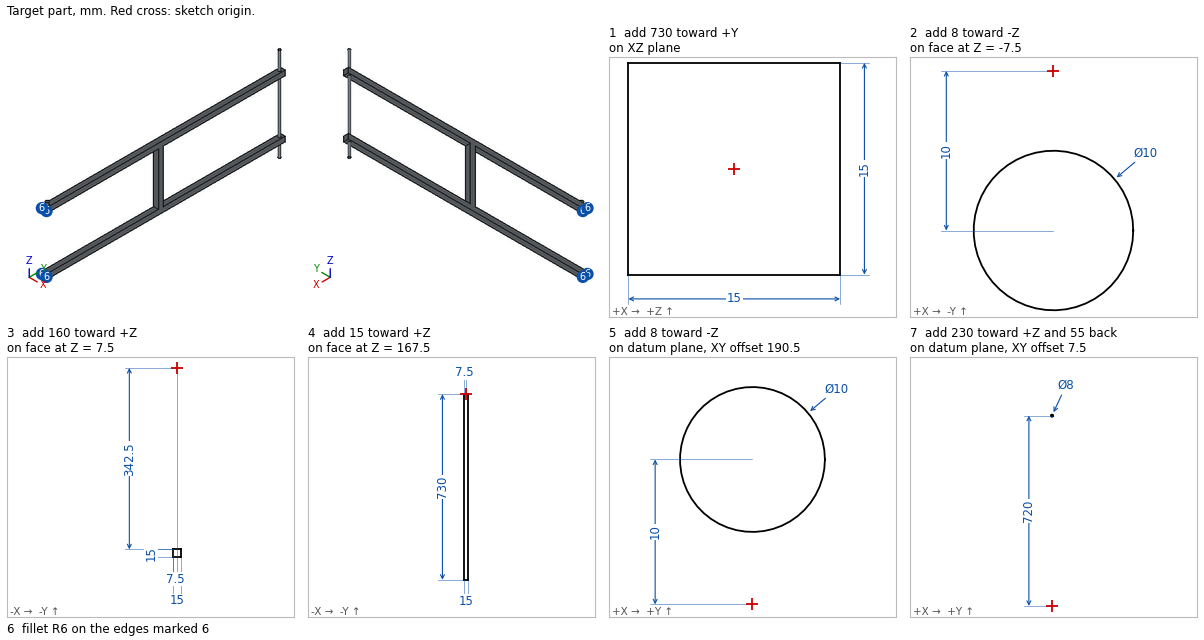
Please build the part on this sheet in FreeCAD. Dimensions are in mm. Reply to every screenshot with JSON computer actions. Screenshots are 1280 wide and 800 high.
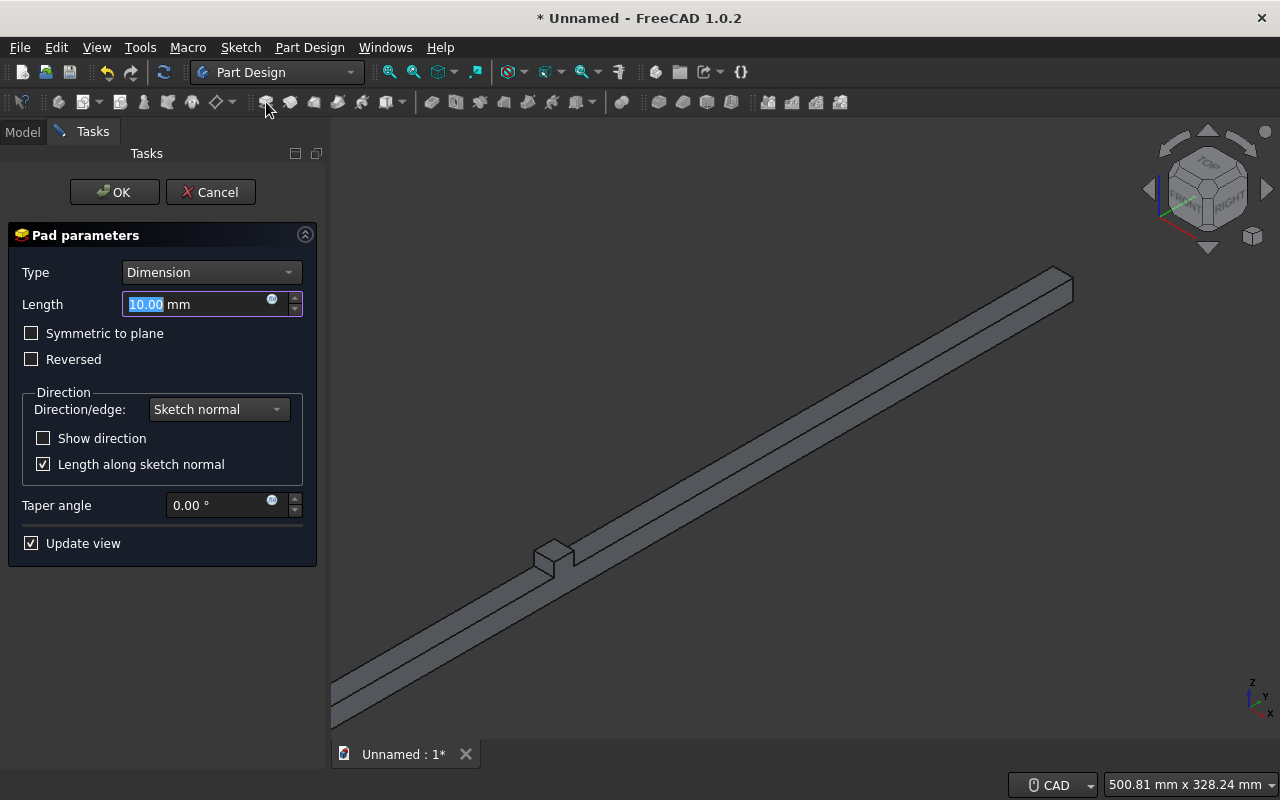
{"action": "type", "text": "160"}
{"action": "key", "text": "Tab"}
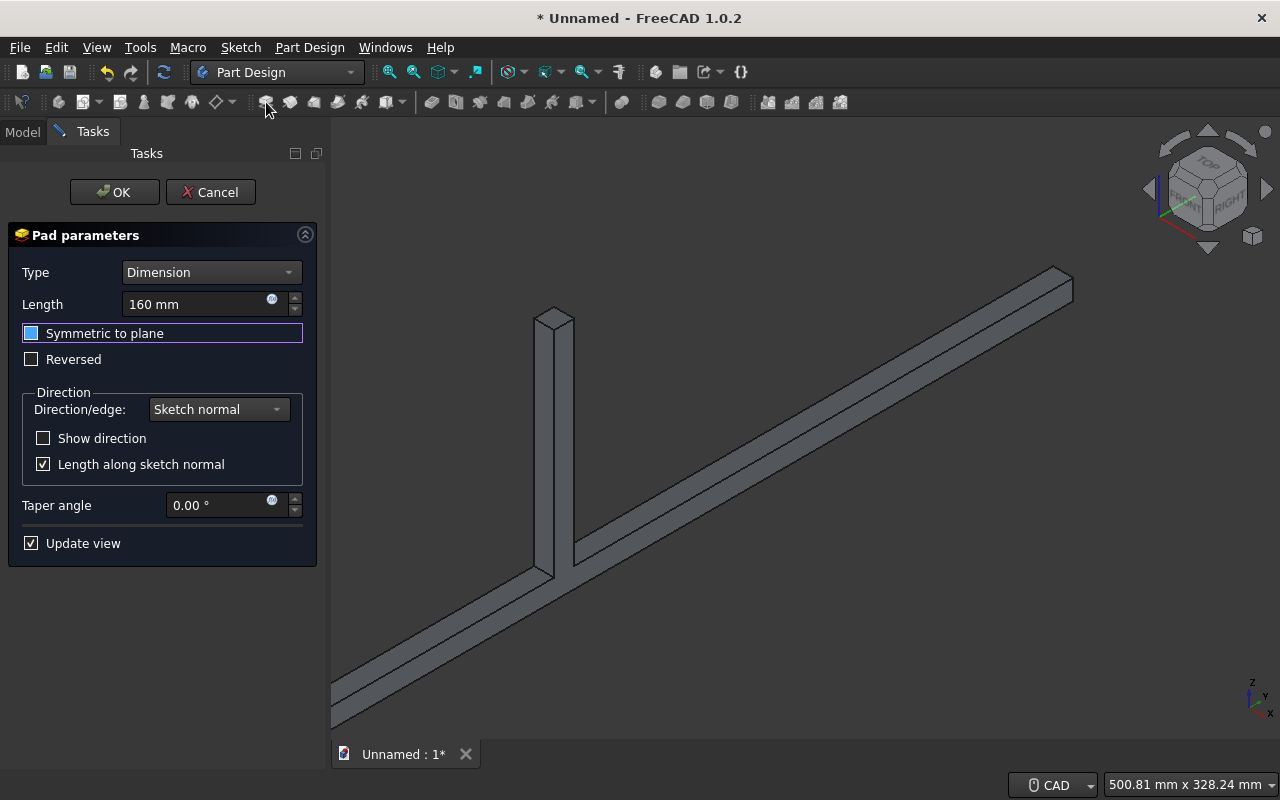
{"action": "left_click", "coordinate": [115, 192]}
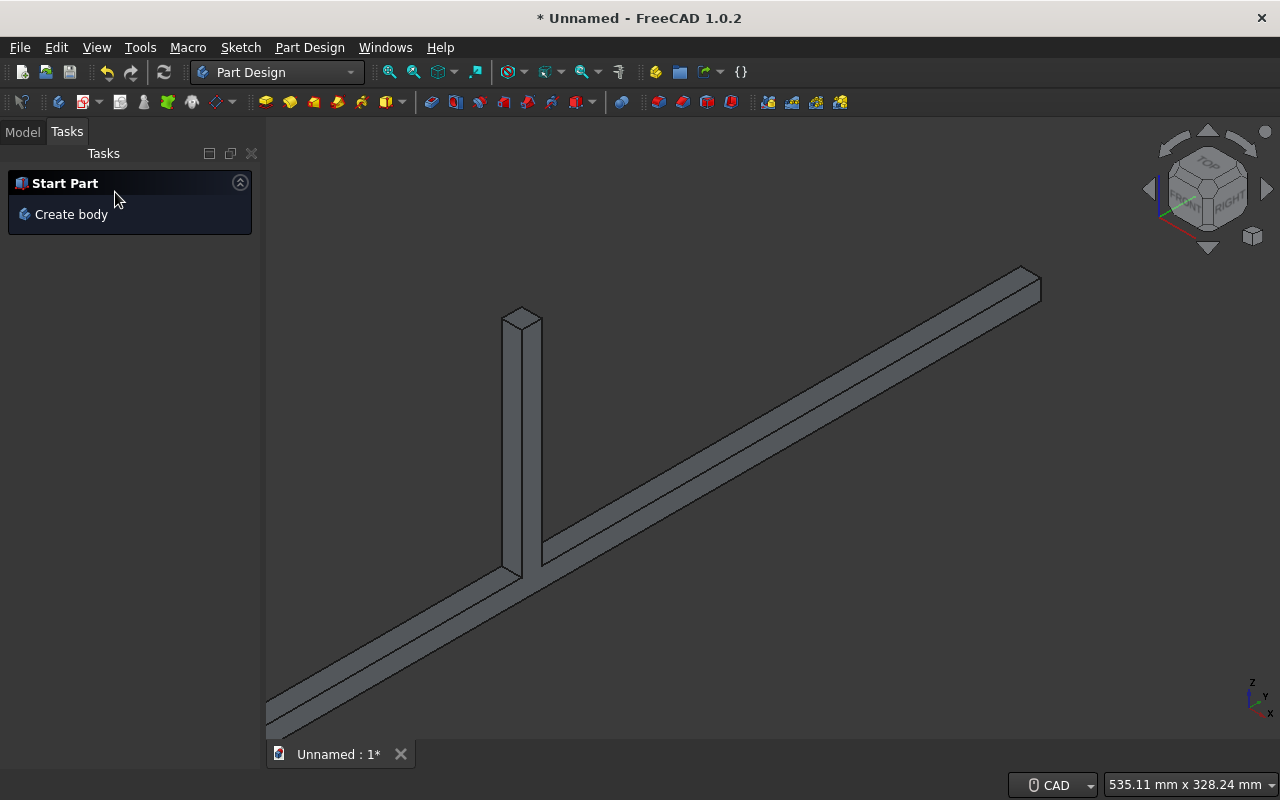
{"action": "left_click", "coordinate": [390, 72]}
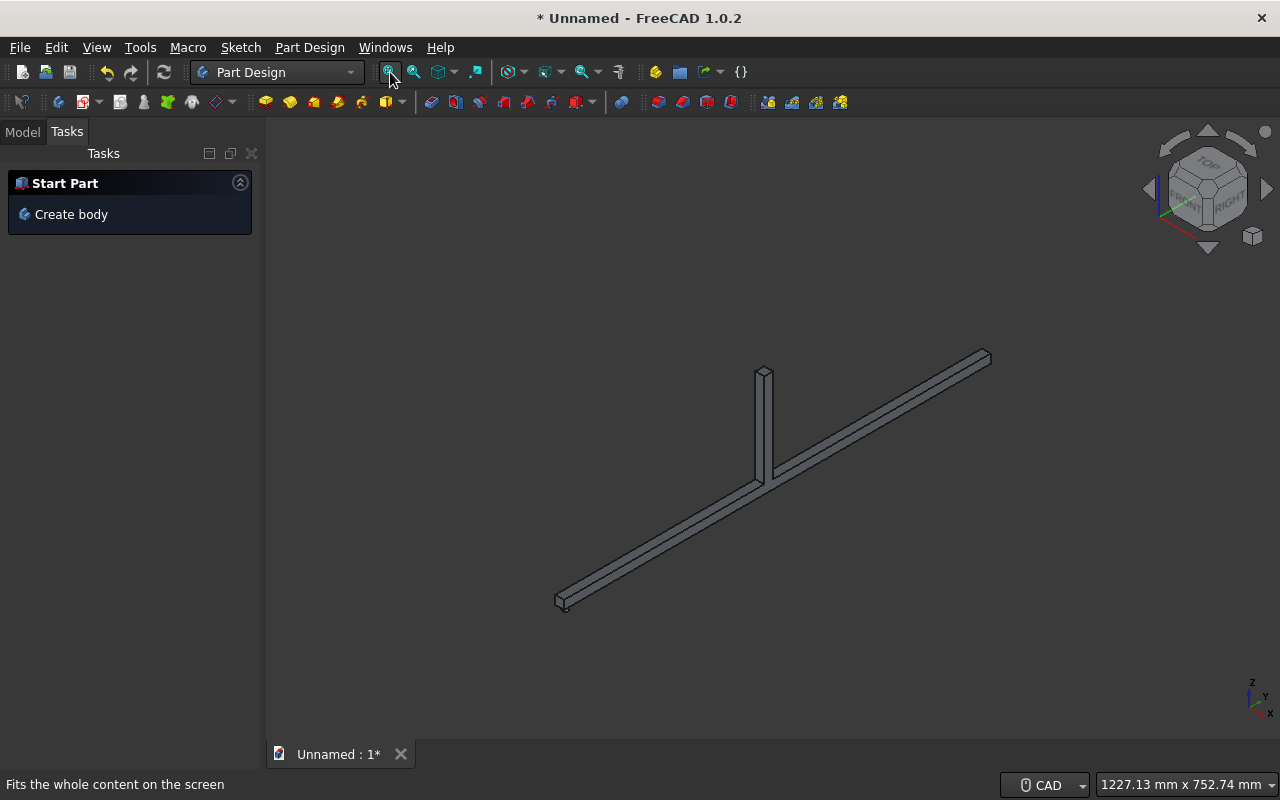
{"action": "scroll", "coordinate": [764, 370], "scroll_direction": "up", "scroll_amount": 4}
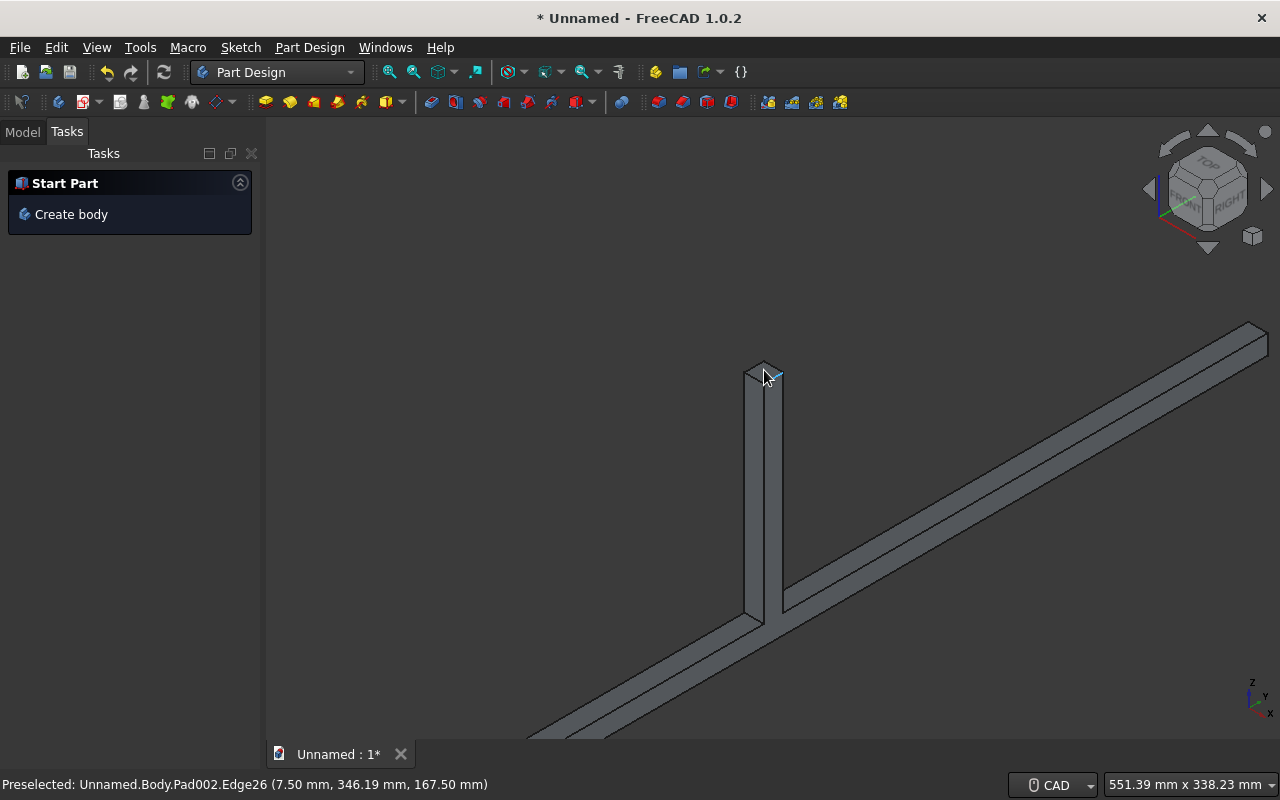
{"action": "left_click", "coordinate": [764, 371]}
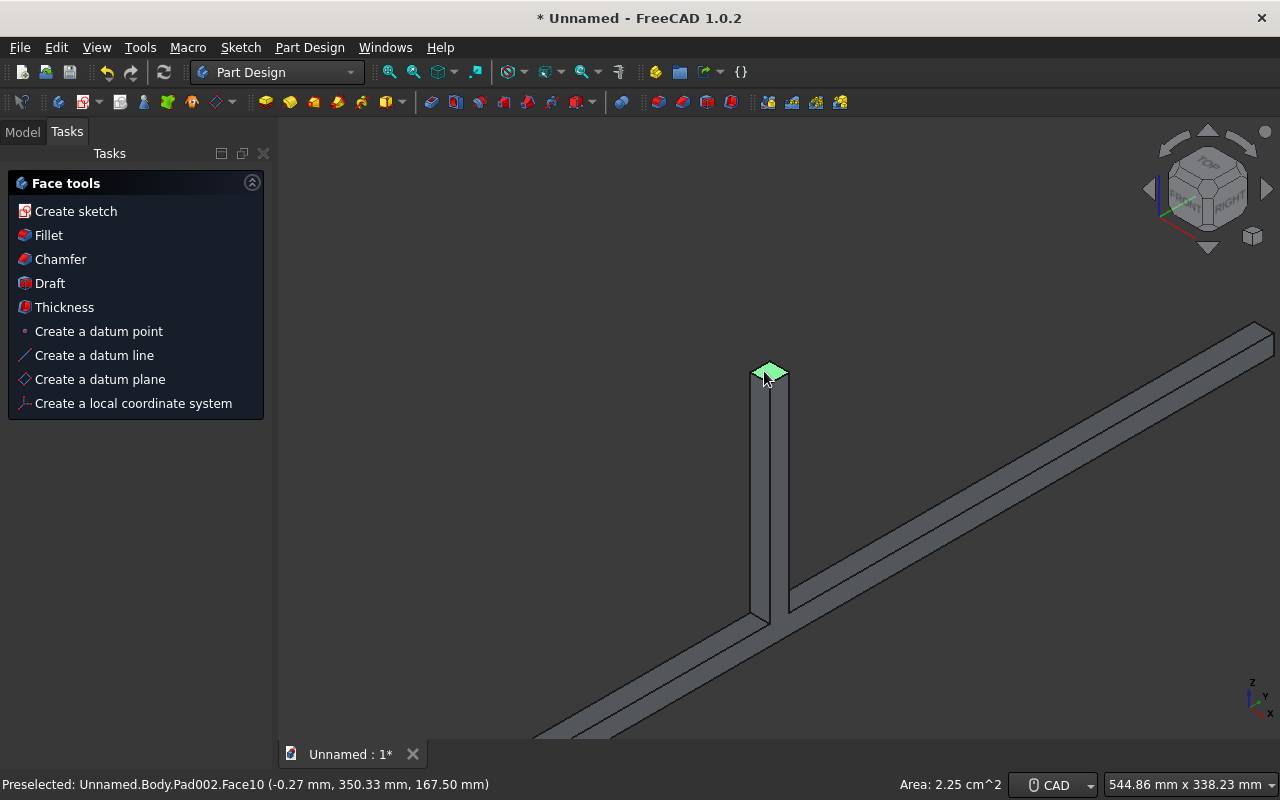
{"action": "left_click", "coordinate": [84, 102]}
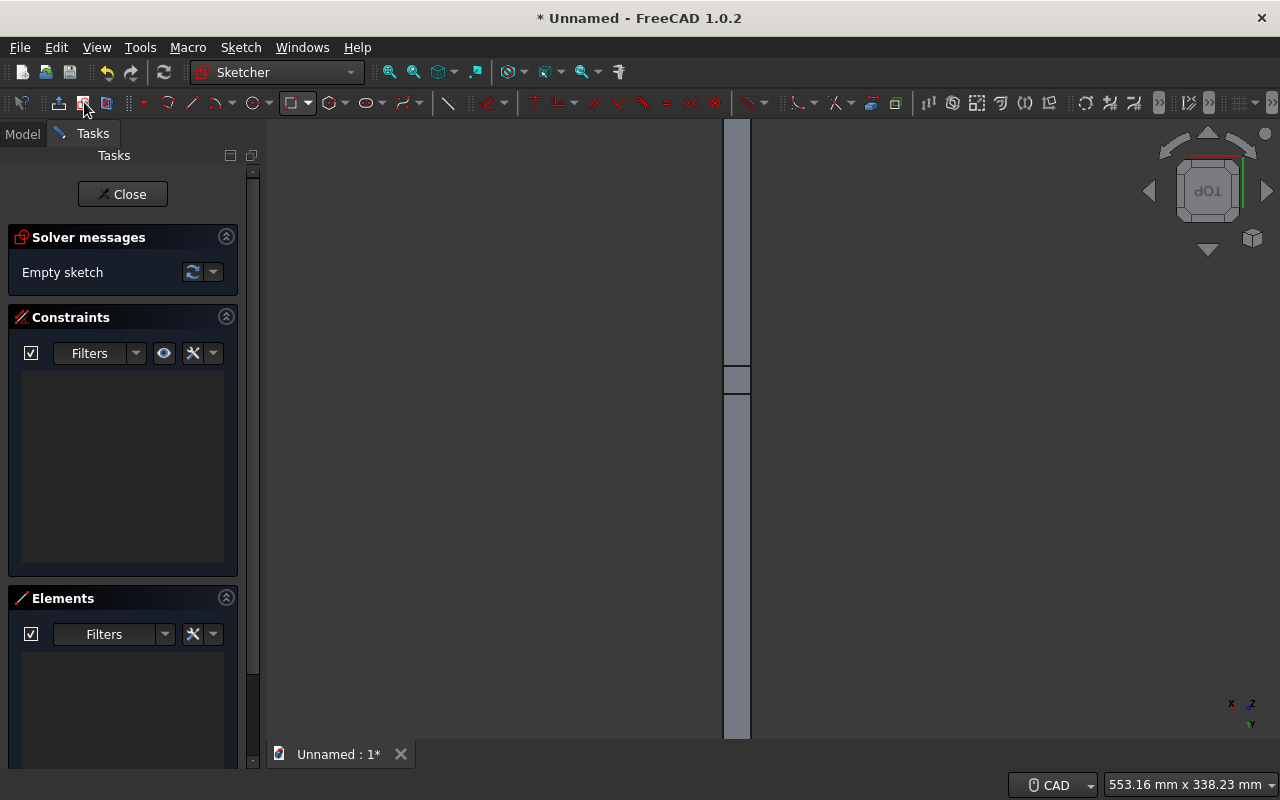
{"action": "scroll", "coordinate": [691, 438], "scroll_direction": "down", "scroll_amount": 6}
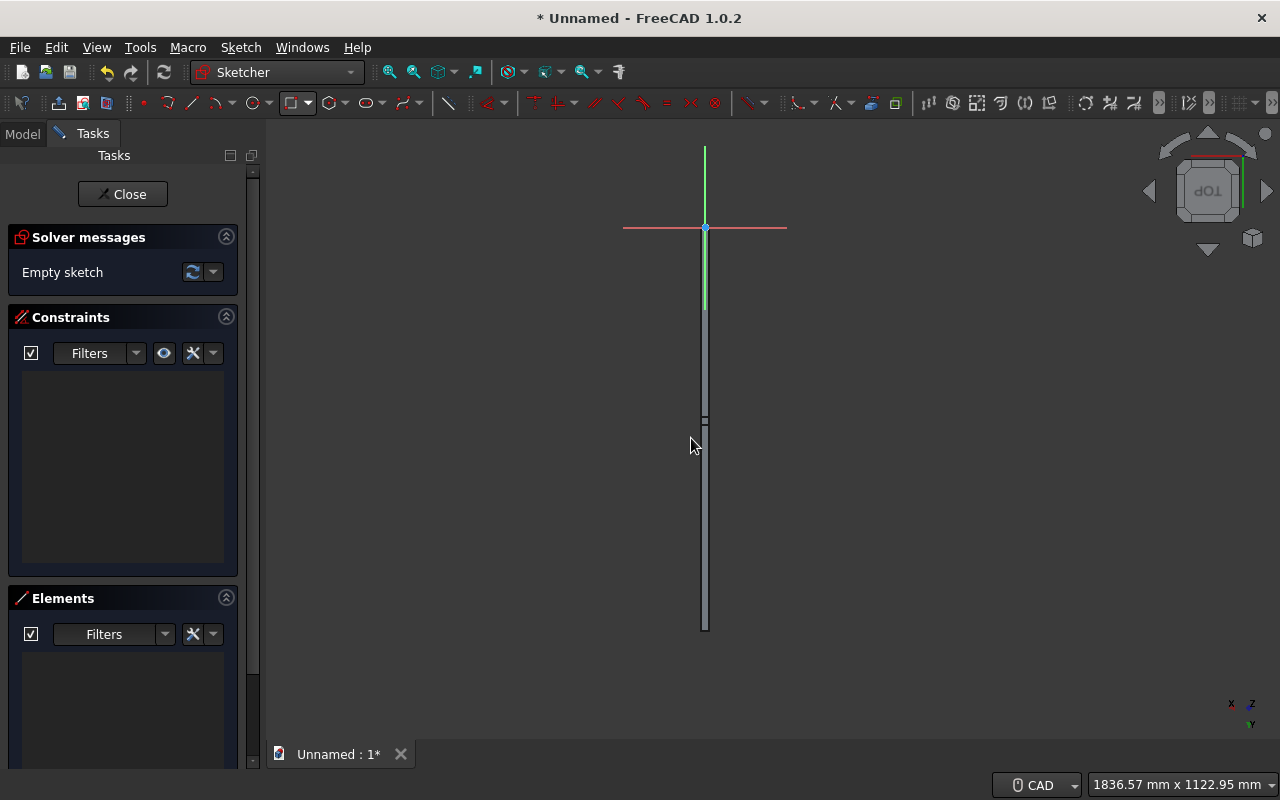
{"action": "left_click", "coordinate": [292, 104]}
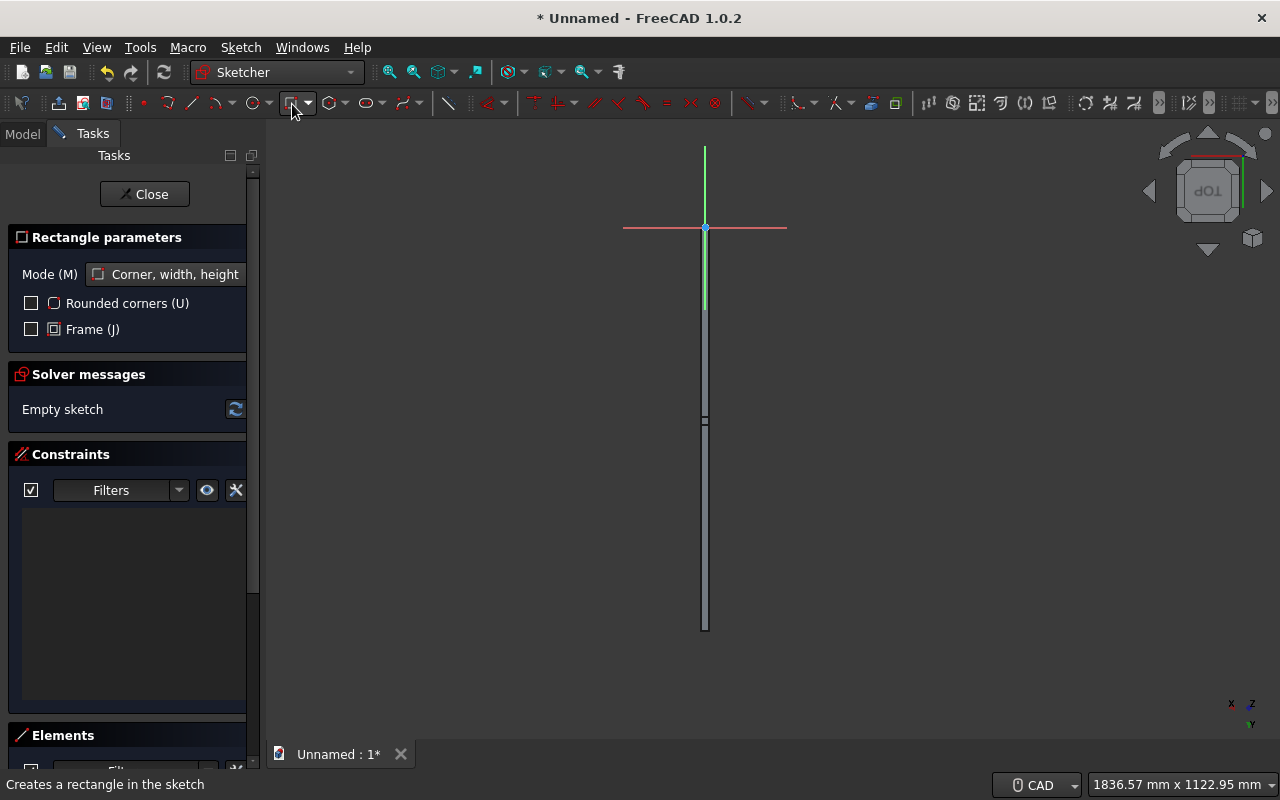
{"action": "scroll", "coordinate": [701, 228], "scroll_direction": "up", "scroll_amount": 7}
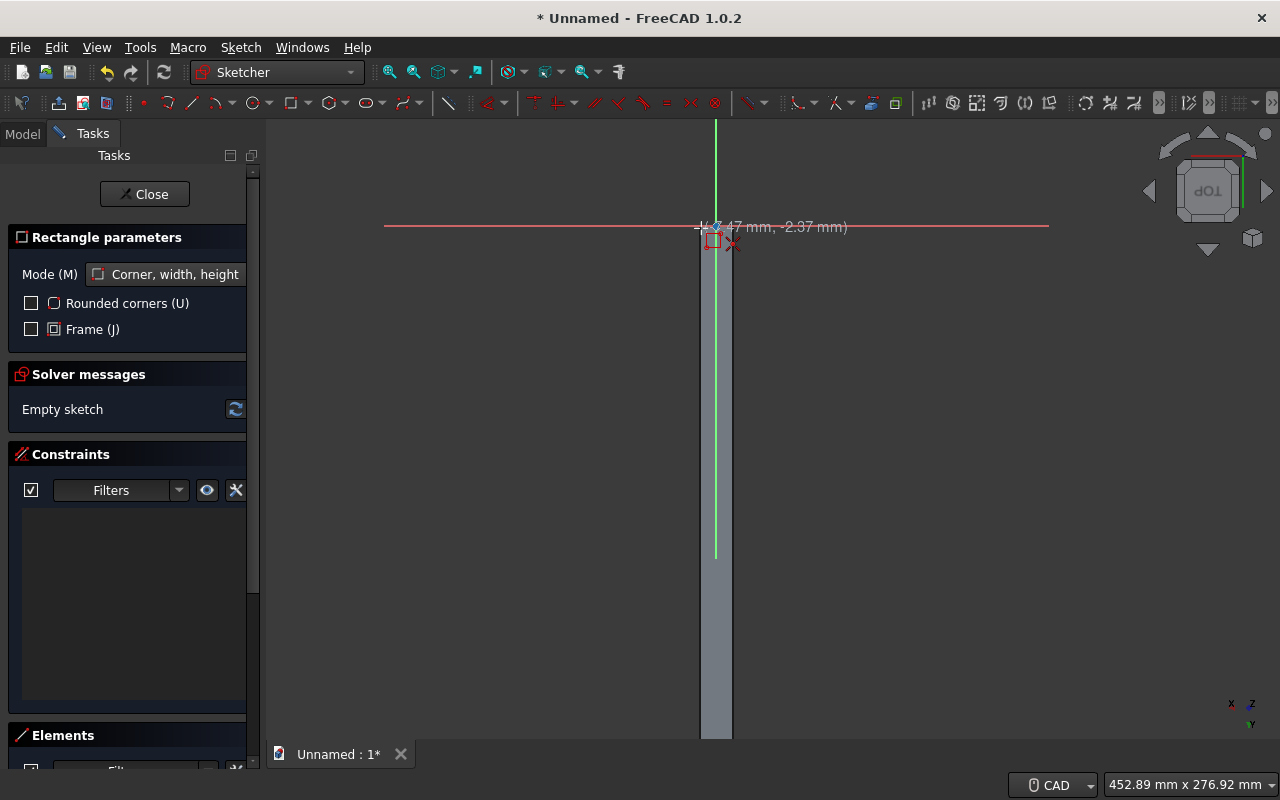
{"action": "left_click", "coordinate": [700, 226]}